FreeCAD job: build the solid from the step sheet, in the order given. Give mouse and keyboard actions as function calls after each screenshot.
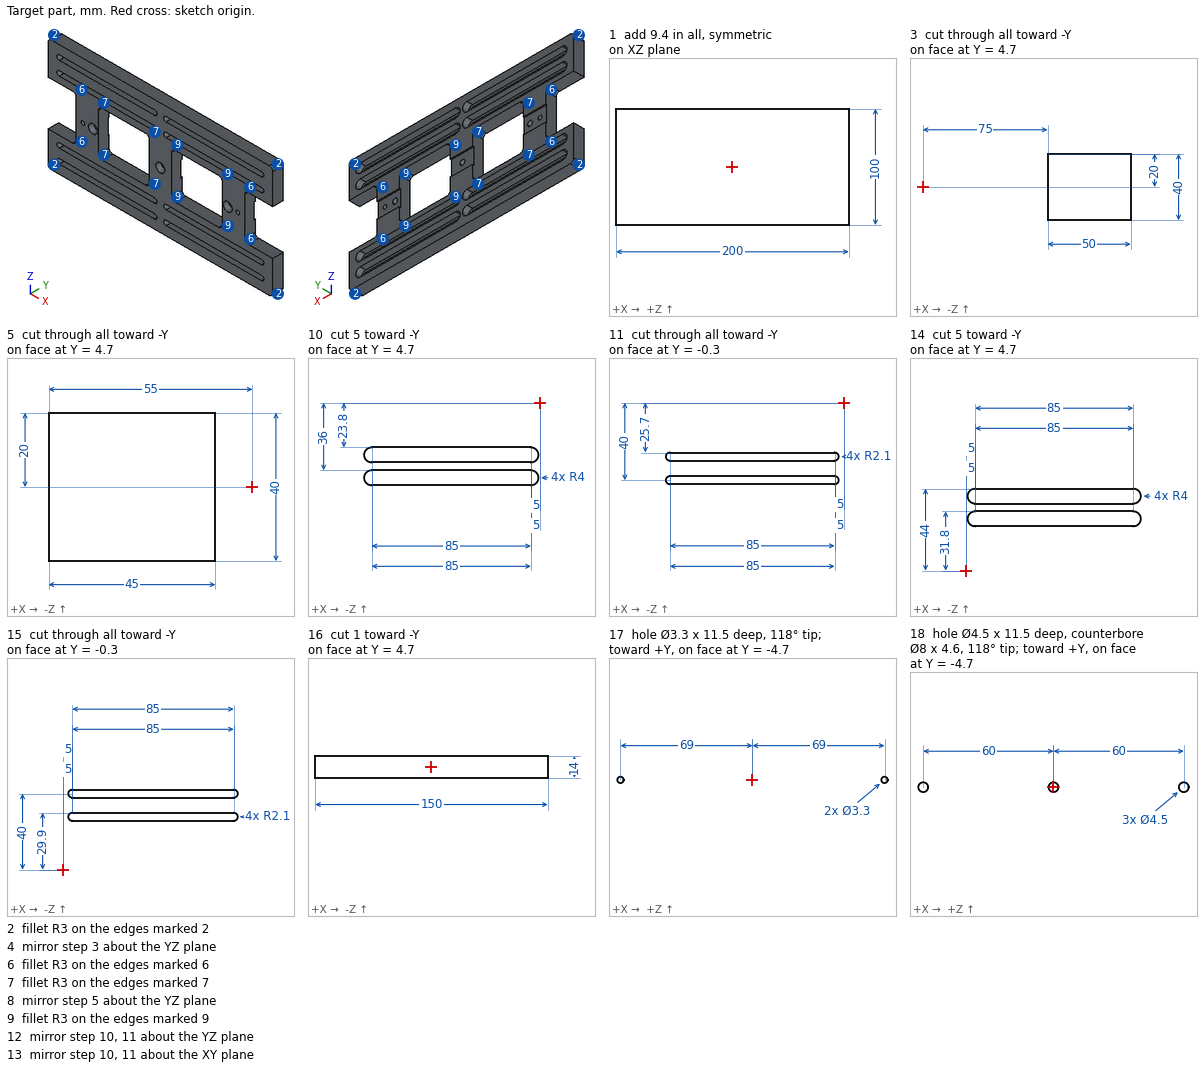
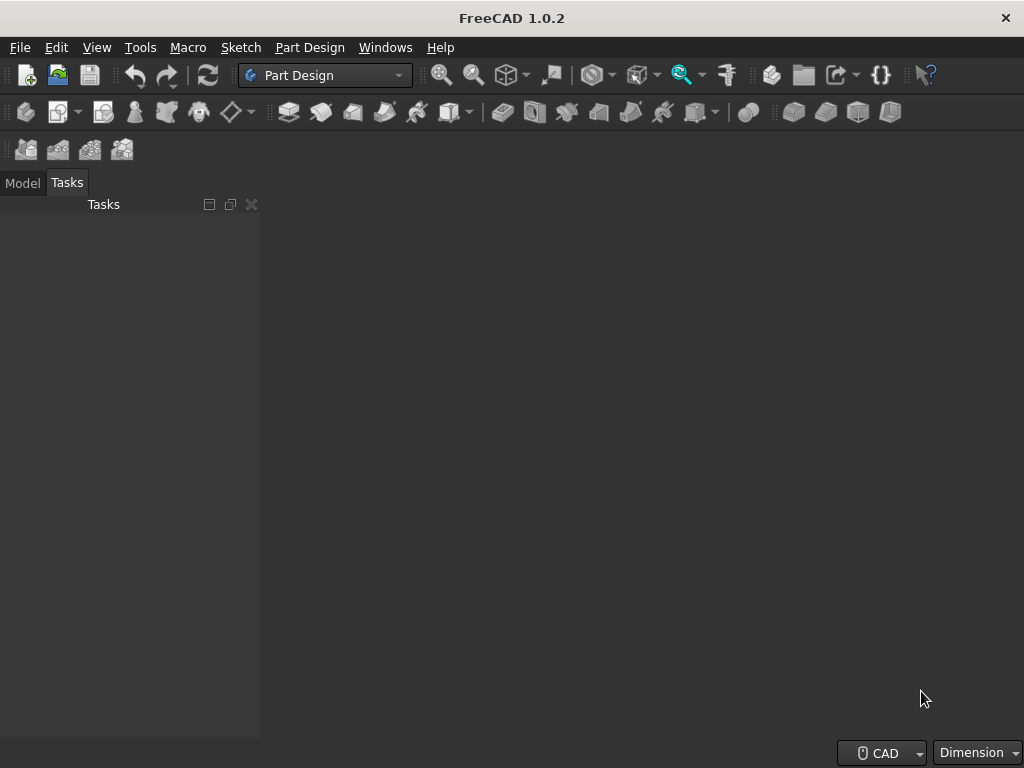
key(ctrl+n)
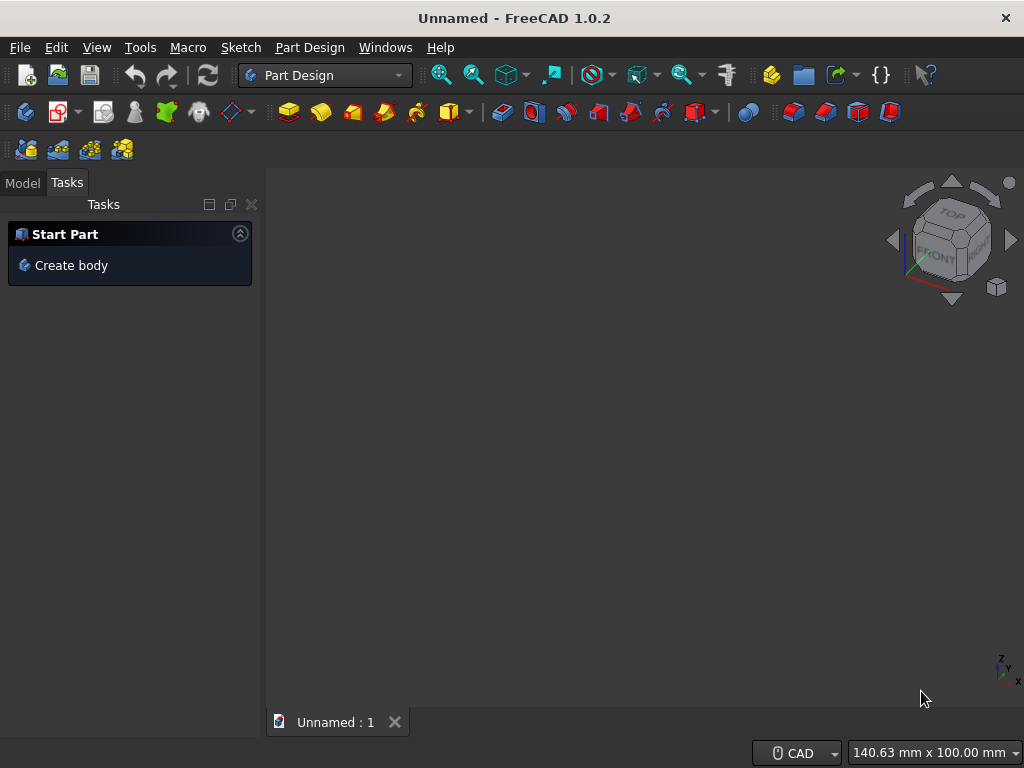
click(58, 112)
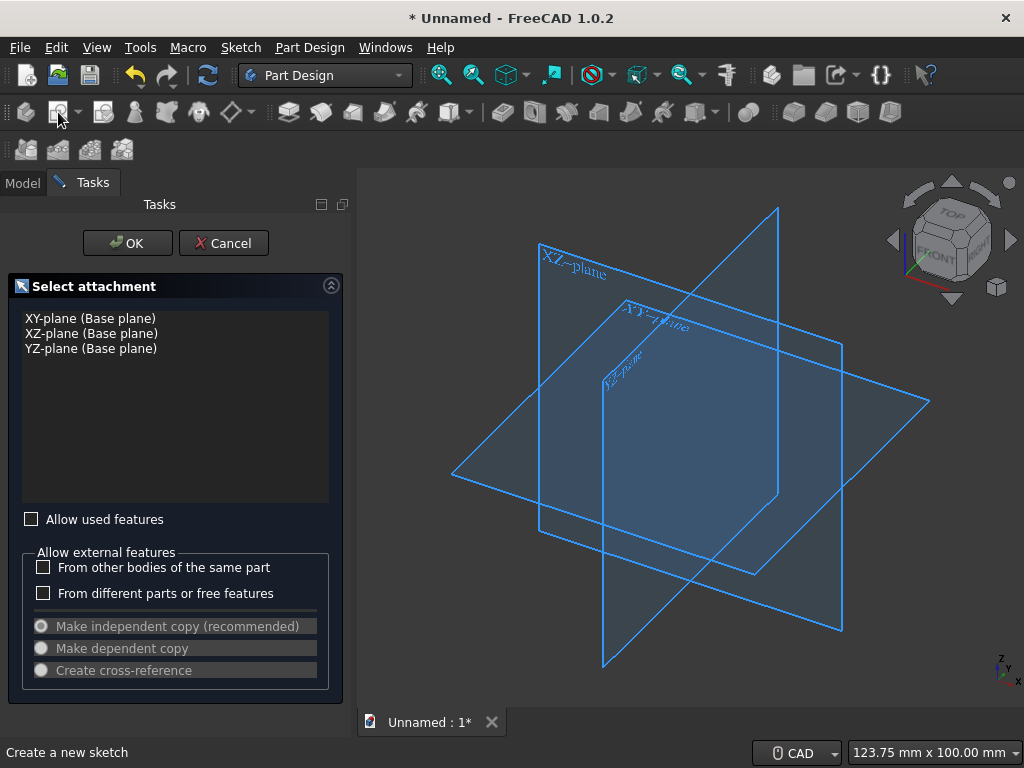
click(82, 334)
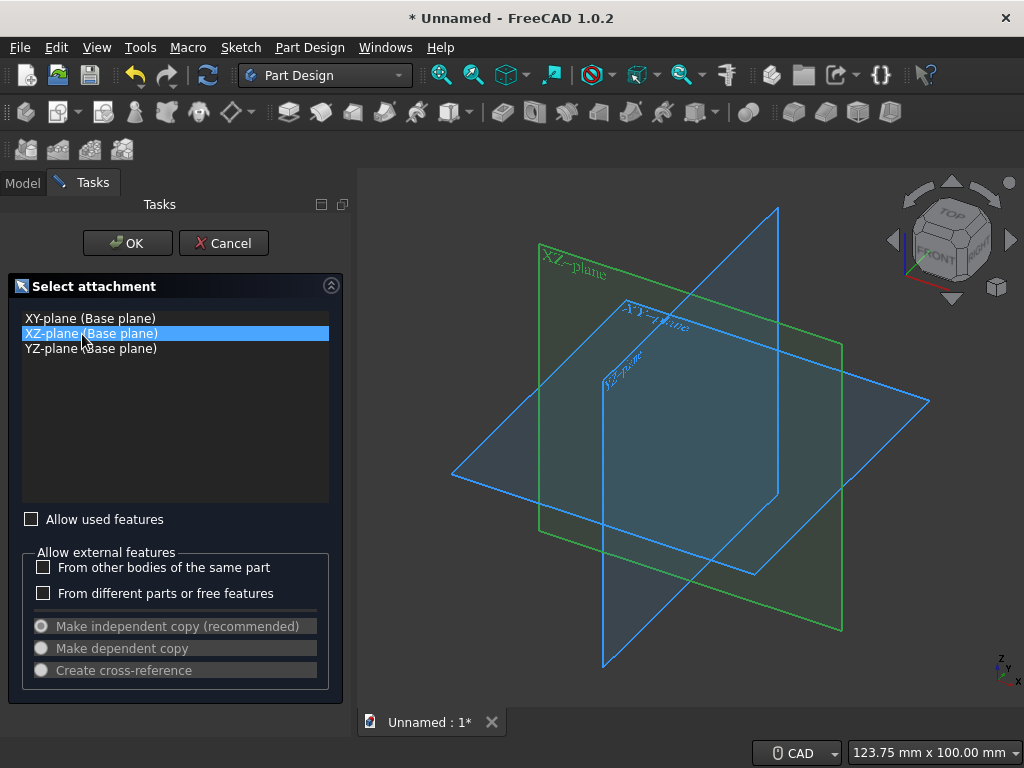
click(128, 243)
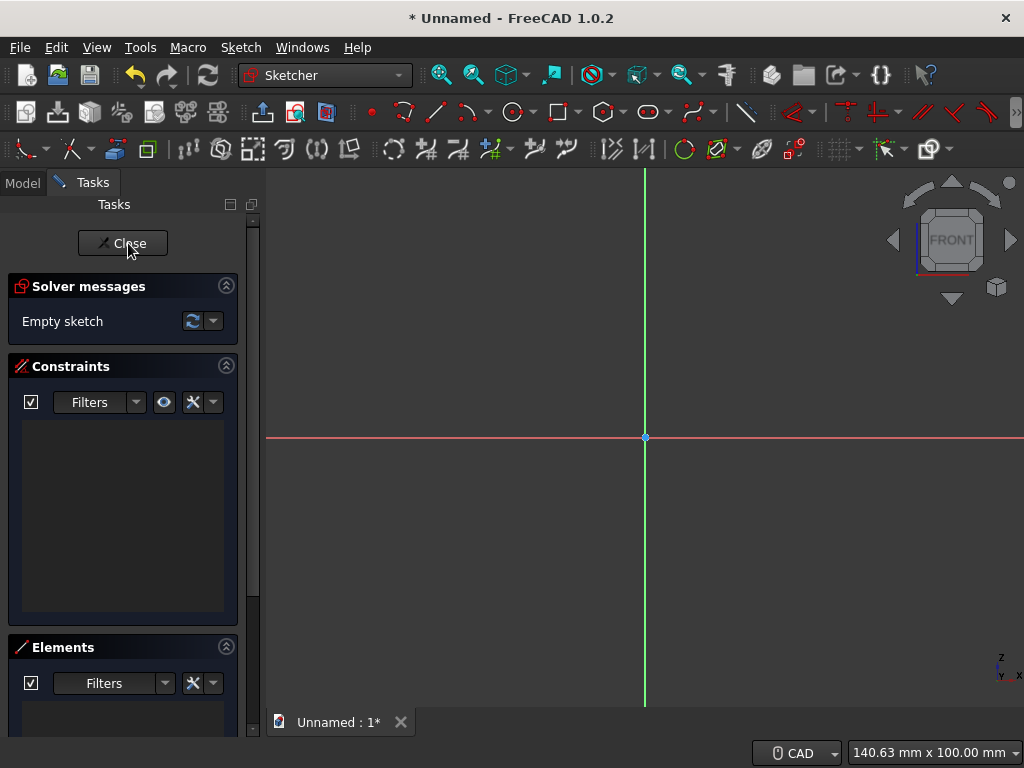
scroll(537, 438, down, 5)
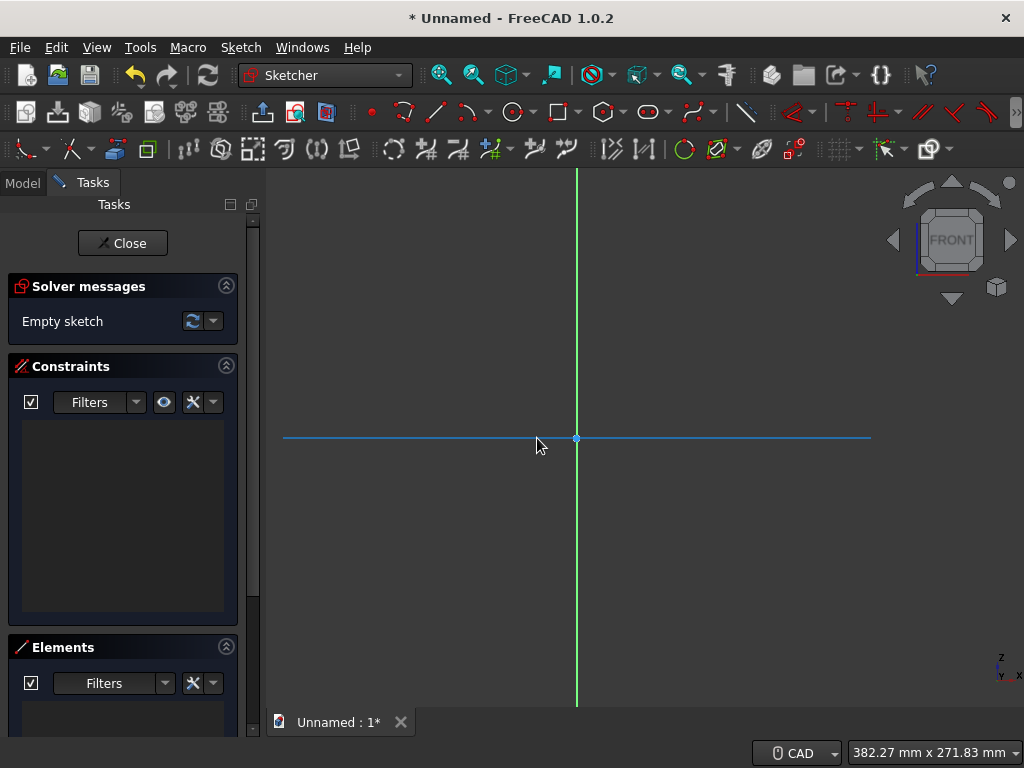
key(g)
key(v)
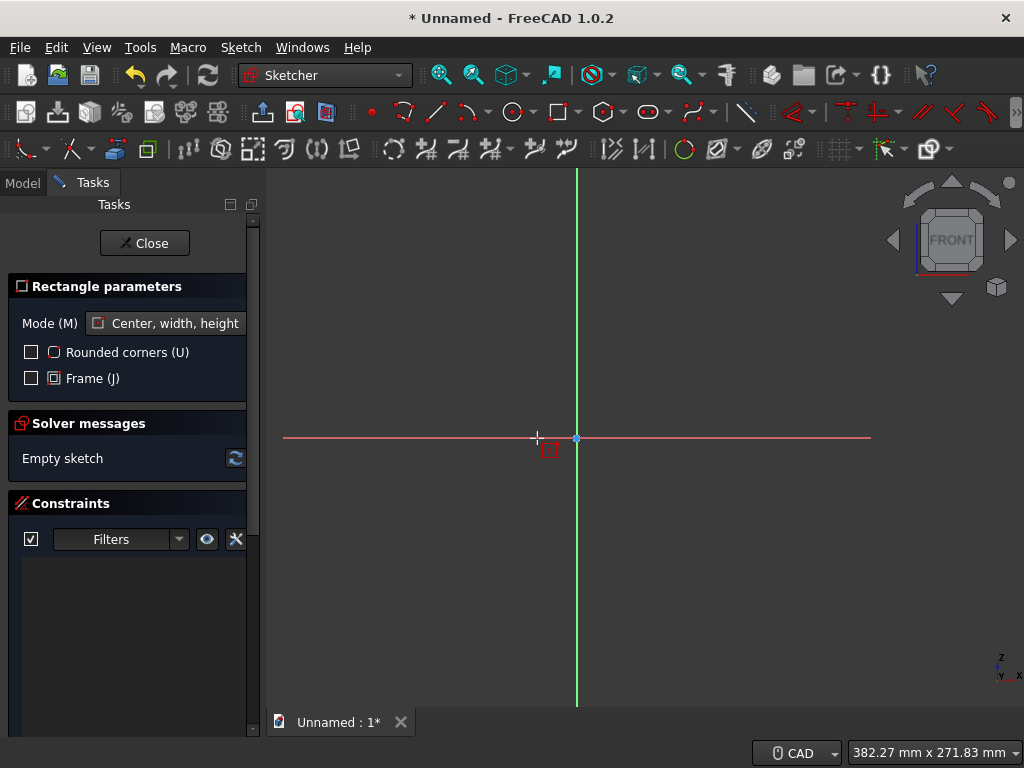
click(577, 438)
move(775, 339)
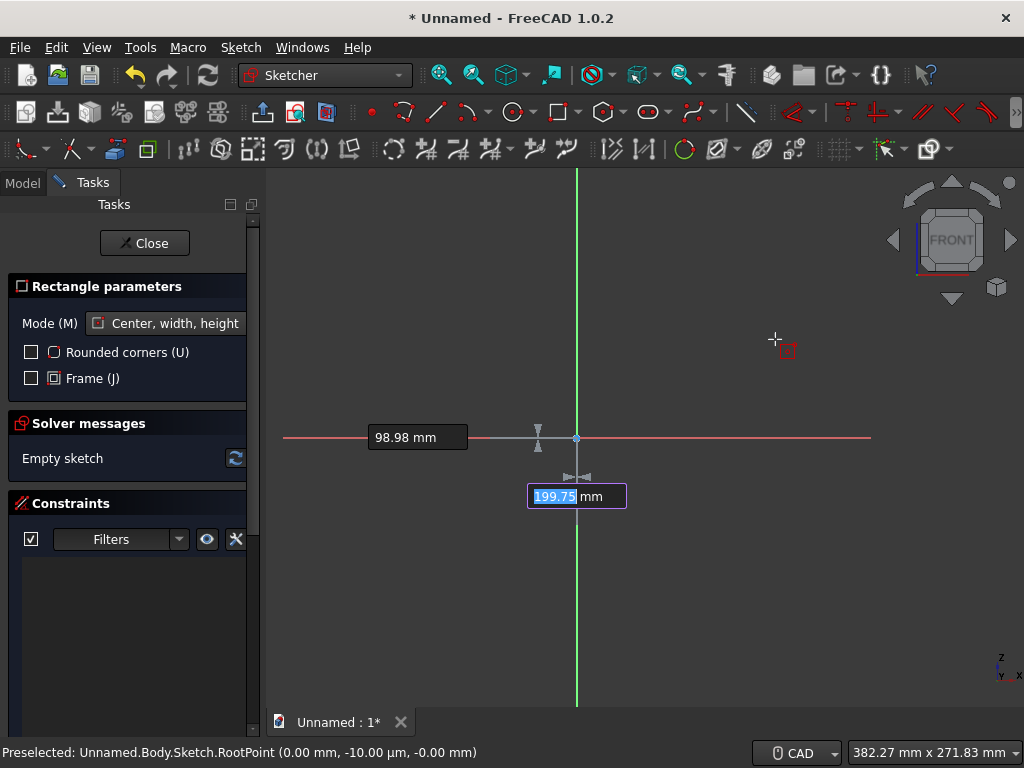
text(200)
key(Tab)
text(100)
key(Return)
key(Escape)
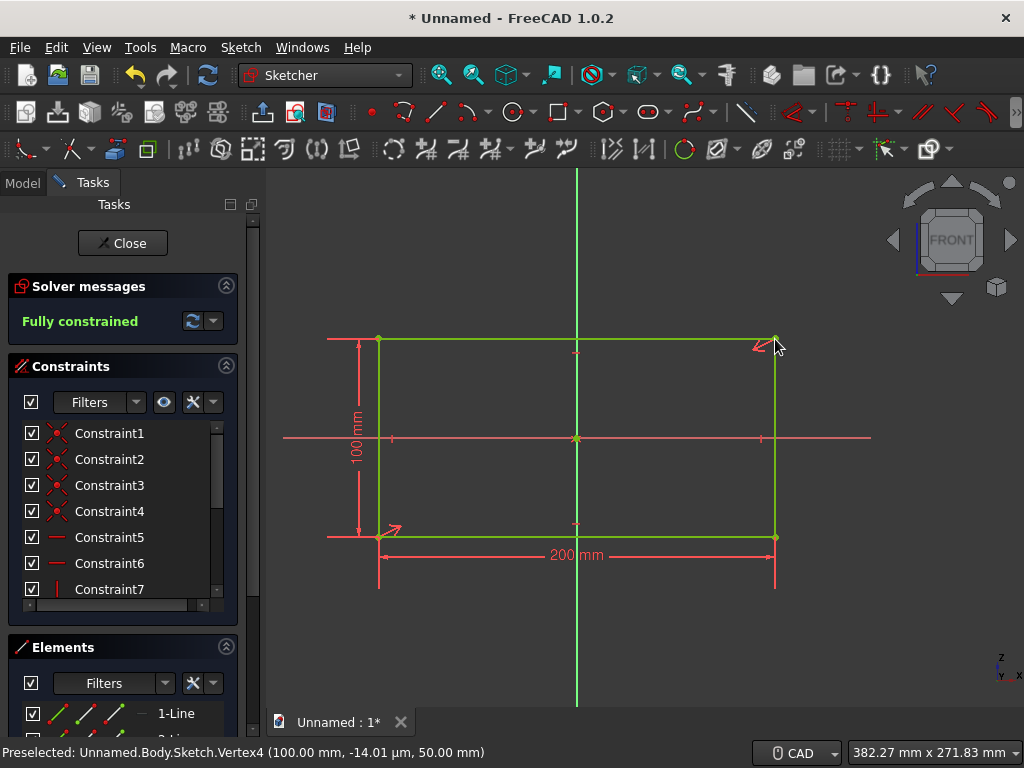
click(123, 243)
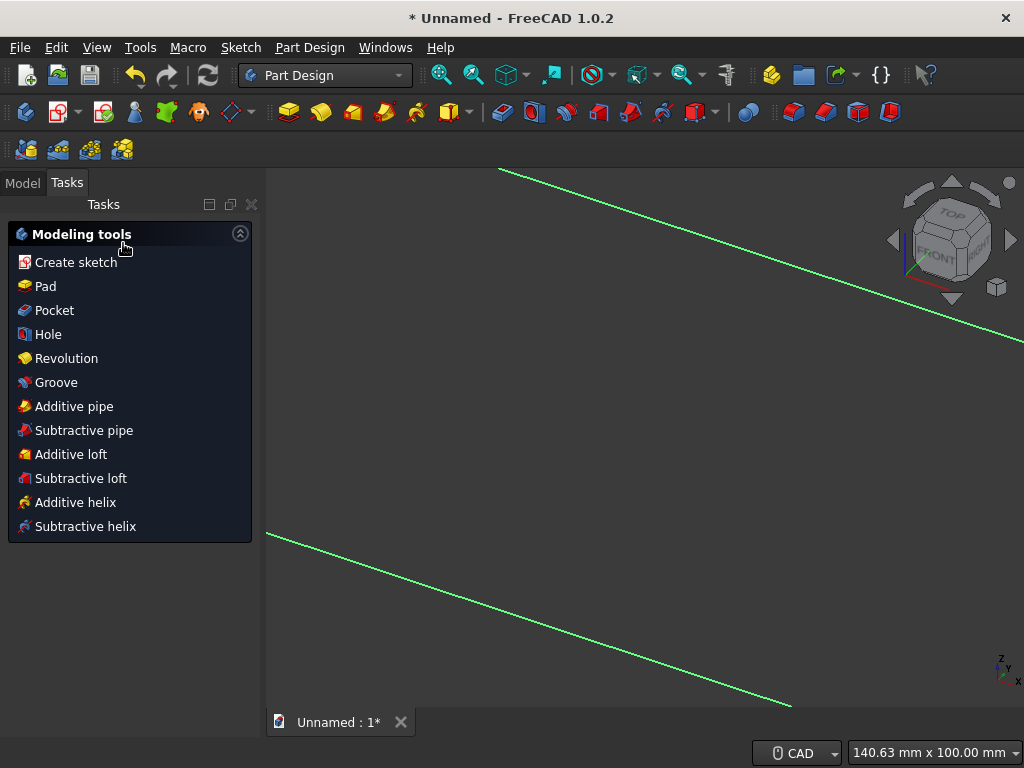
click(290, 112)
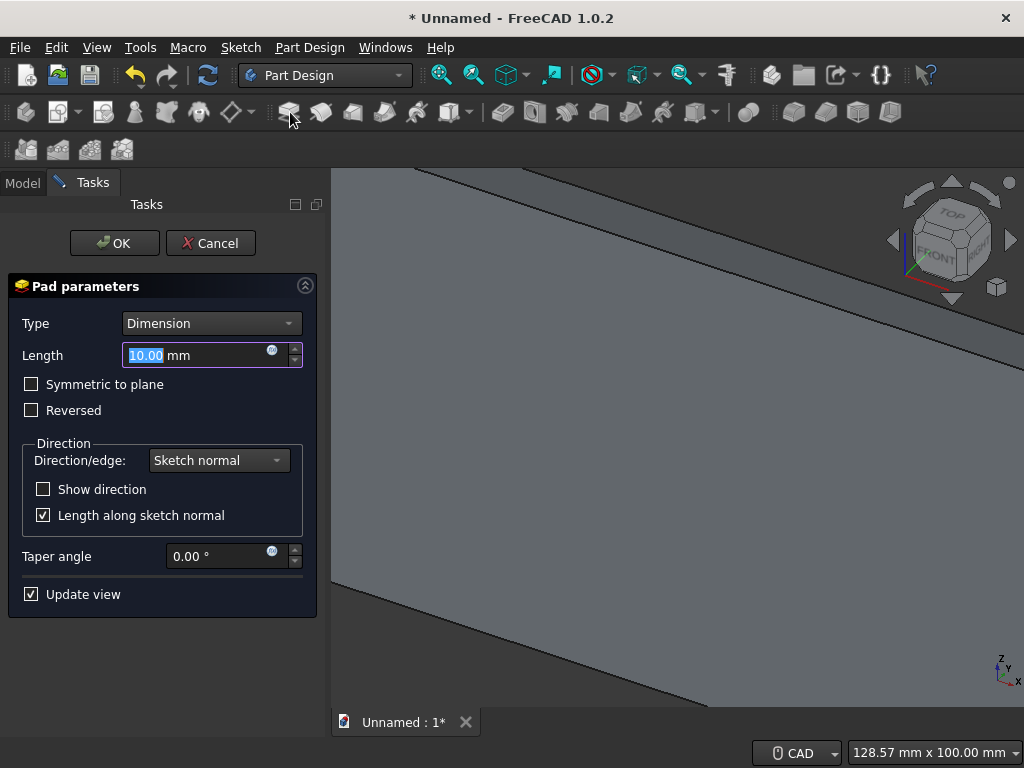
text(9.4)
key(Tab)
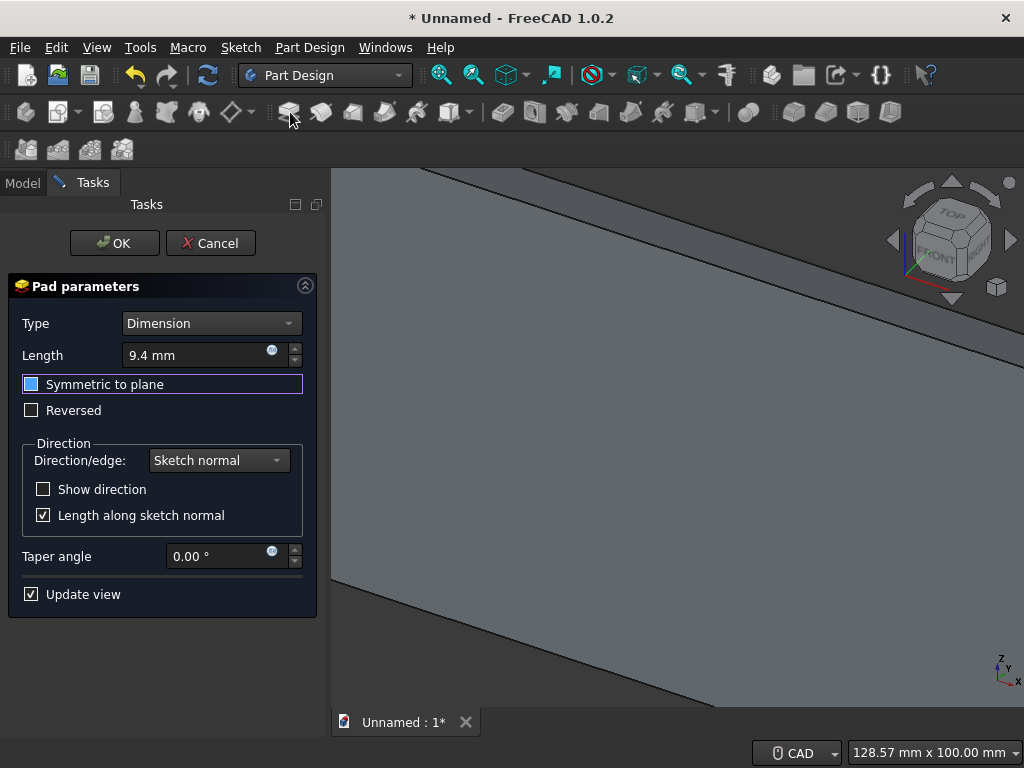
click(30, 384)